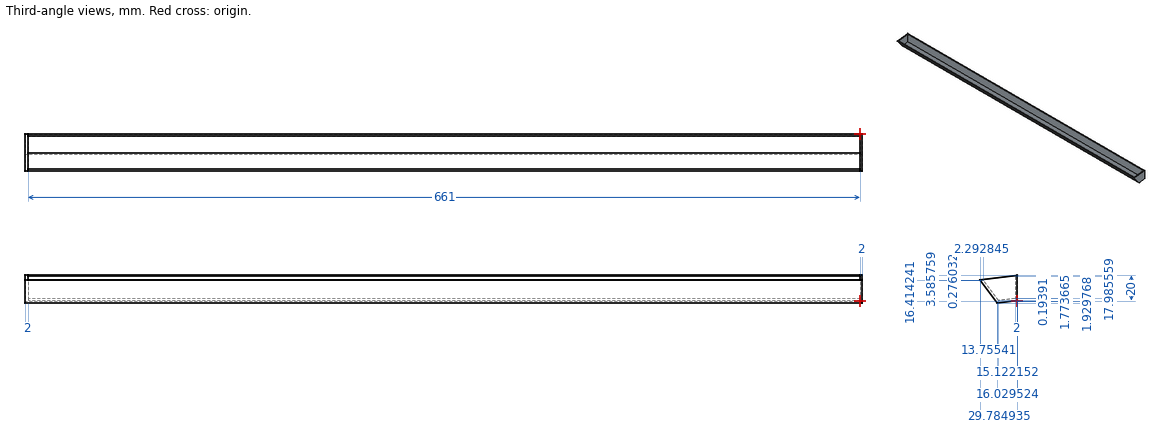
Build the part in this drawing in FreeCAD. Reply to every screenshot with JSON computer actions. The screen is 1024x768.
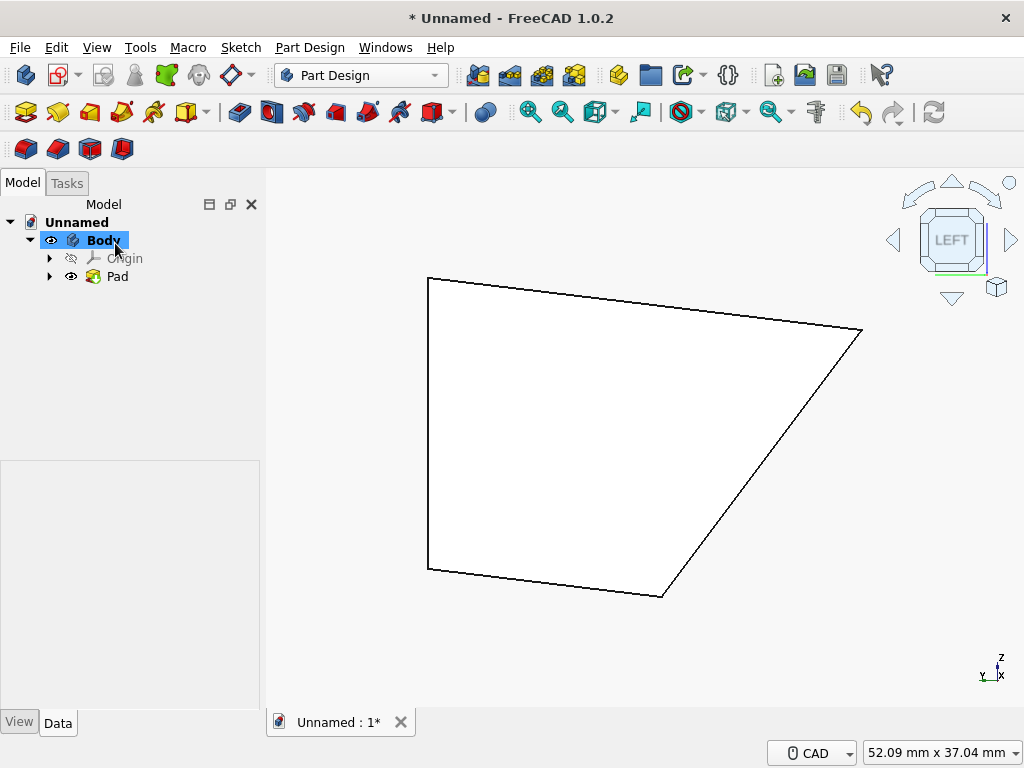
{"action": "left_click", "coordinate": [583, 437]}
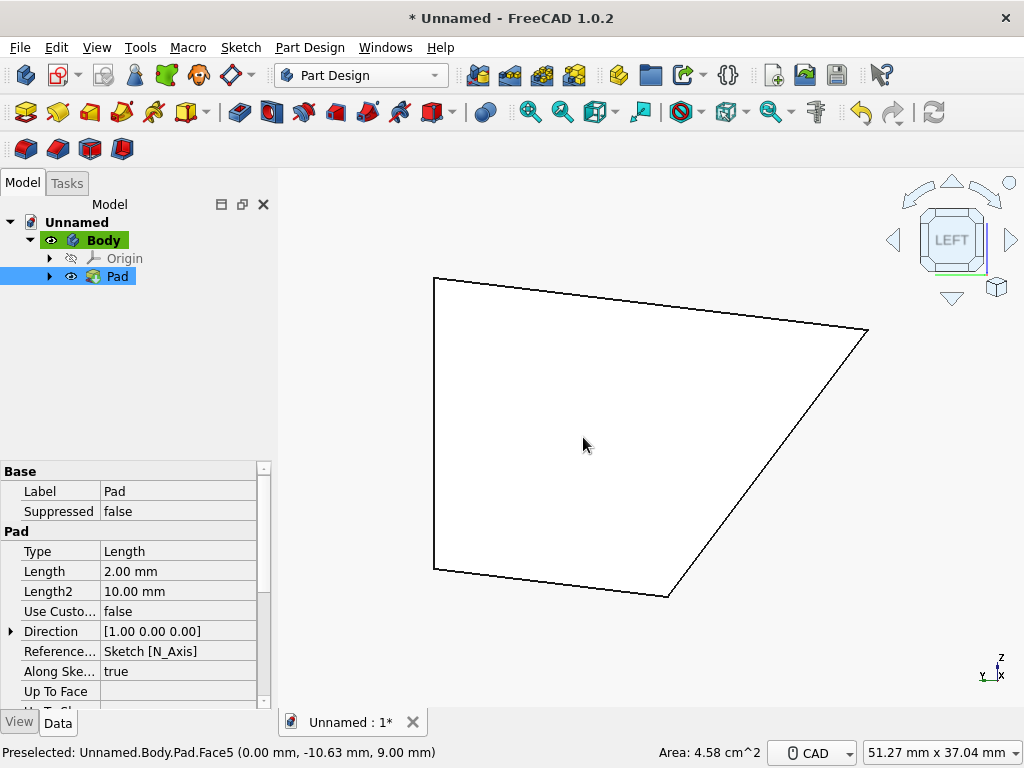
{"action": "left_click", "coordinate": [58, 76]}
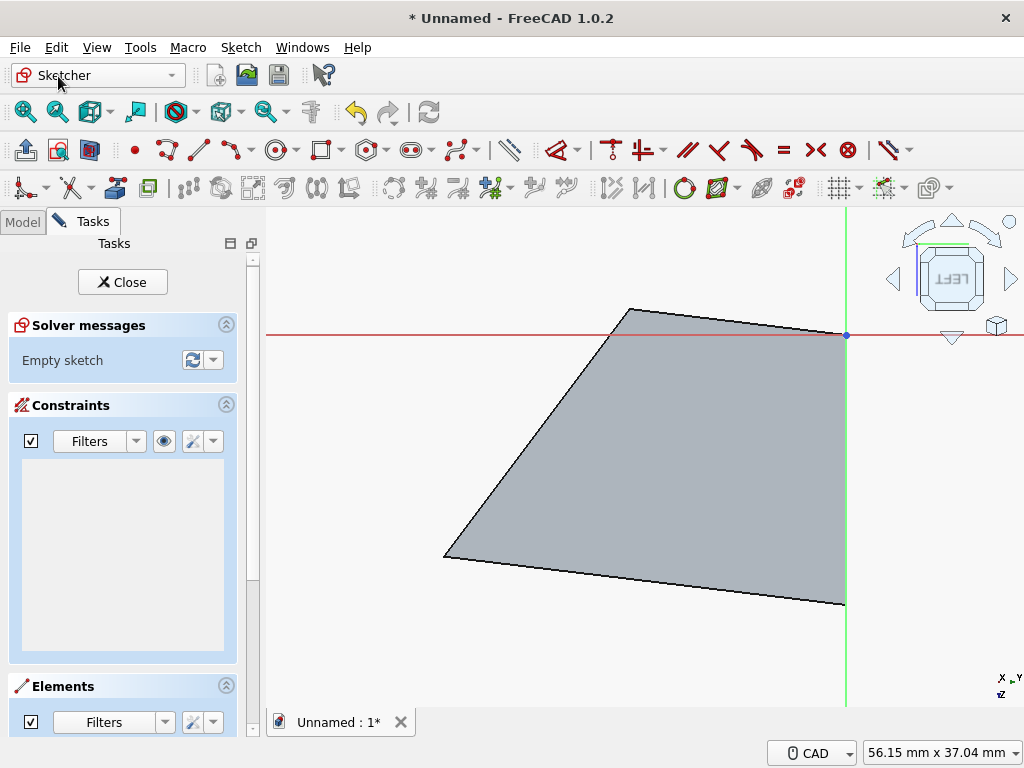
{"action": "scroll", "coordinate": [294, 457], "scroll_direction": "down", "scroll_amount": 1}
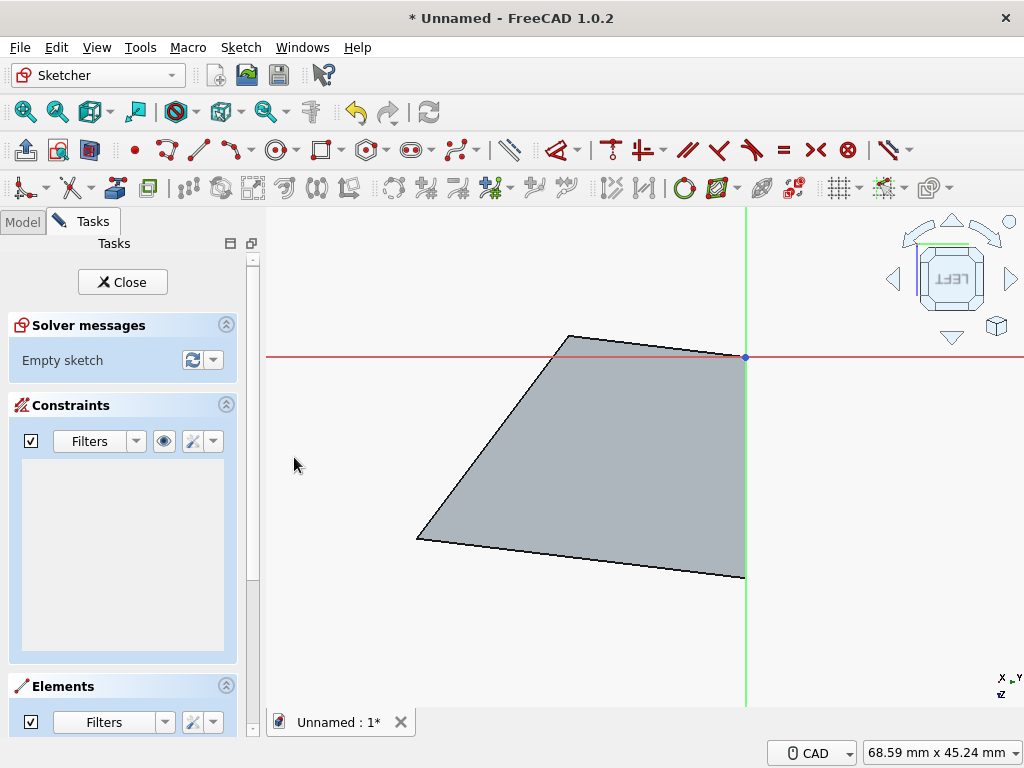
{"action": "left_click", "coordinate": [168, 150]}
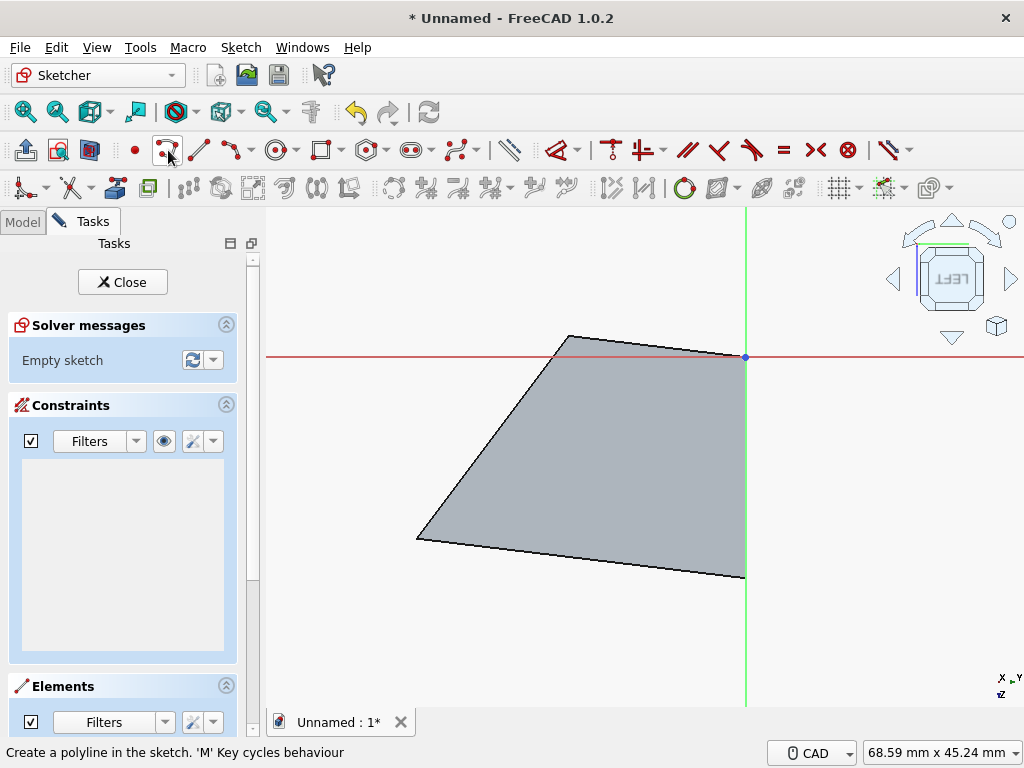
{"action": "left_click", "coordinate": [746, 357]}
{"action": "left_click", "coordinate": [569, 336]}
{"action": "left_click", "coordinate": [417, 539]}
{"action": "left_click", "coordinate": [442, 542]}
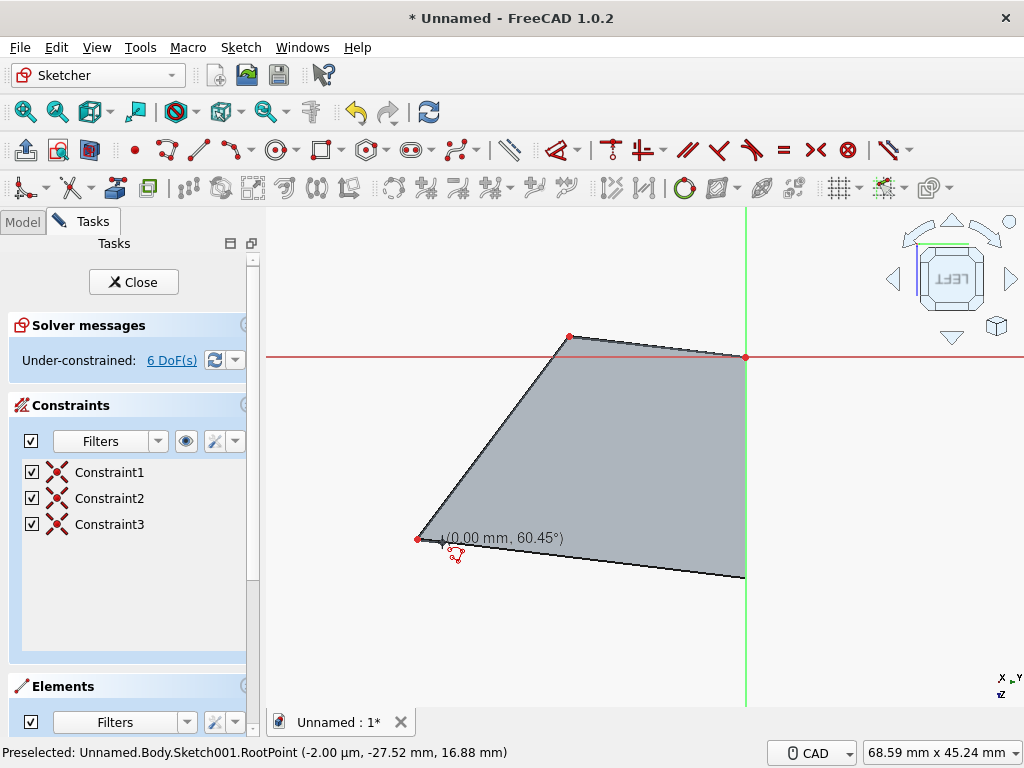
{"action": "scroll", "coordinate": [579, 359], "scroll_direction": "up", "scroll_amount": 11}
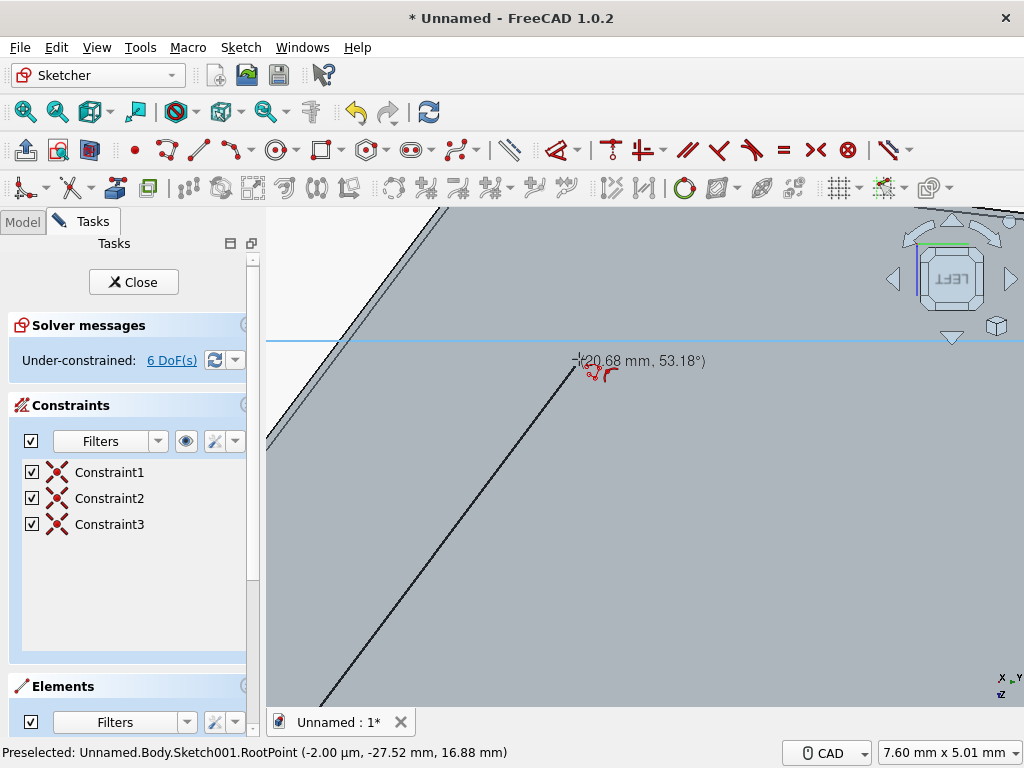
{"action": "left_click", "coordinate": [574, 360]}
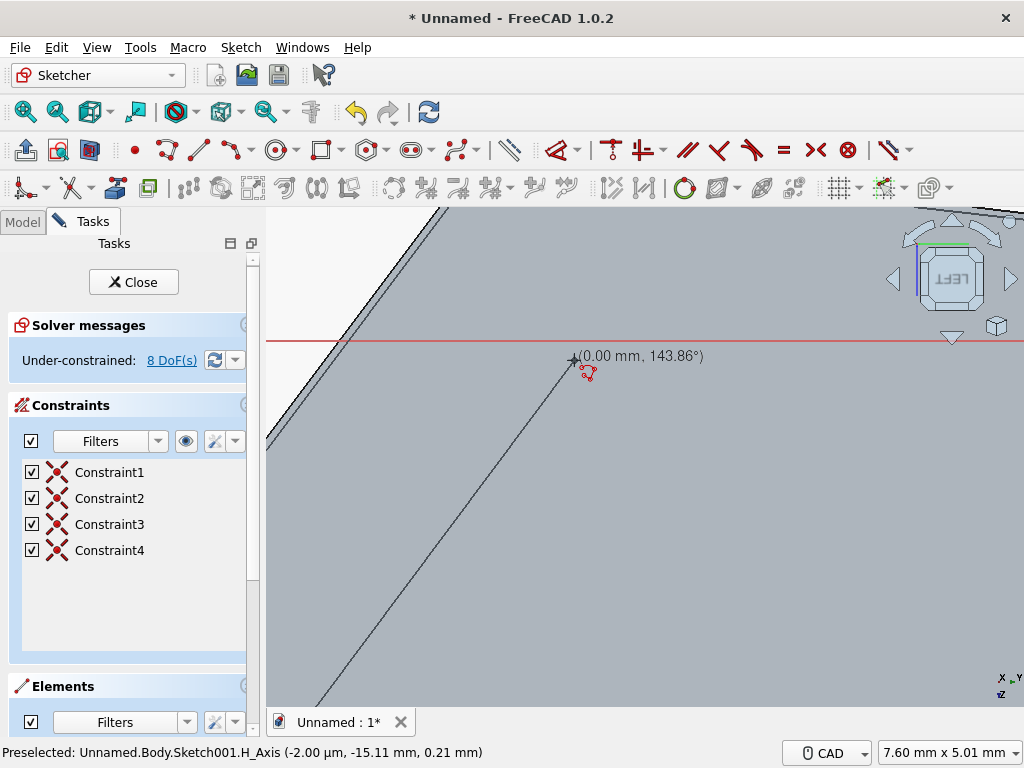
{"action": "scroll", "coordinate": [573, 334], "scroll_direction": "down", "scroll_amount": 10}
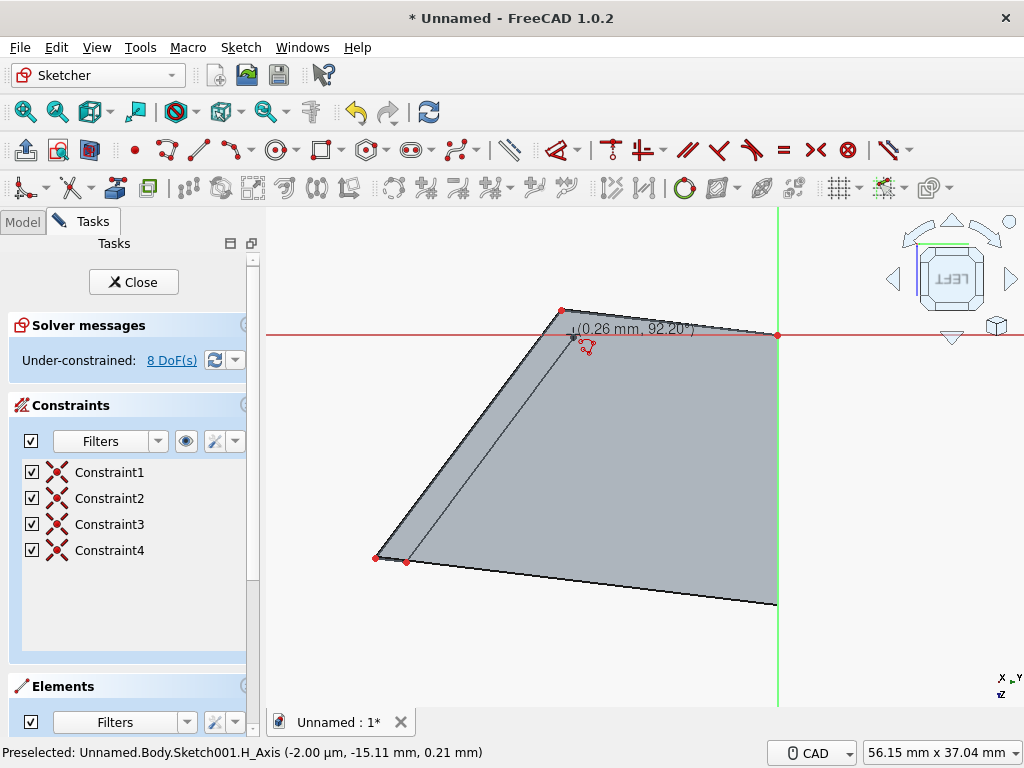
{"action": "left_click", "coordinate": [751, 359]}
{"action": "left_click", "coordinate": [751, 602]}
{"action": "left_click", "coordinate": [769, 605]}
{"action": "left_click", "coordinate": [778, 335]}
{"action": "key", "text": "Escape"}
{"action": "key", "text": "Escape"}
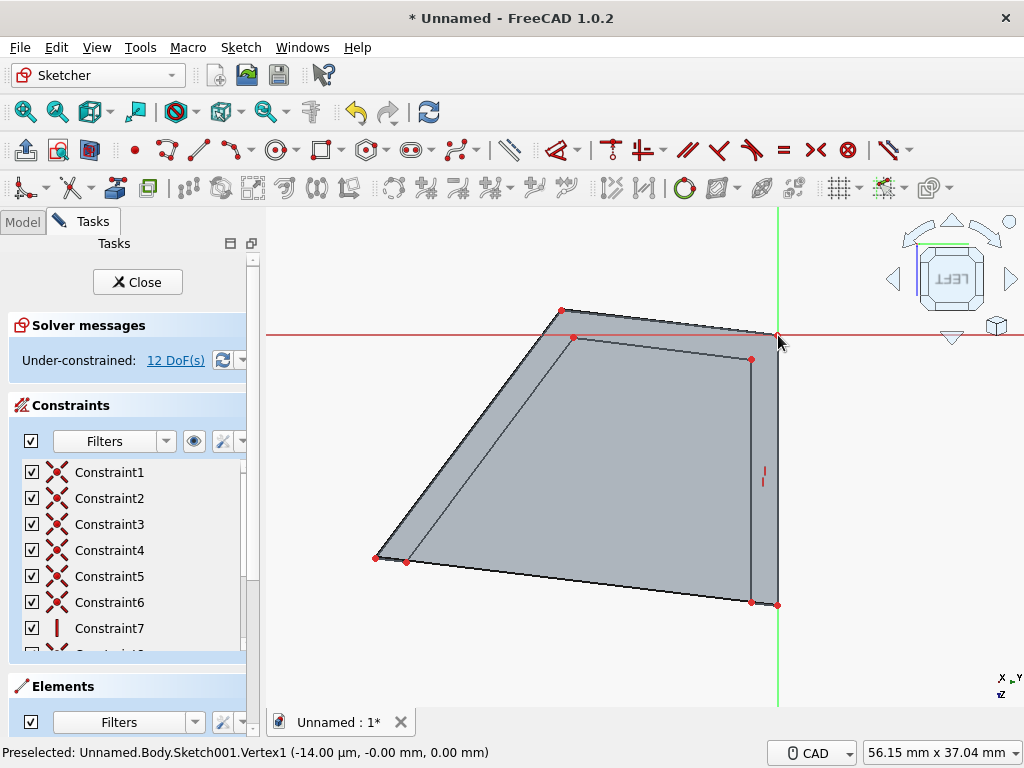
{"action": "left_click", "coordinate": [556, 150]}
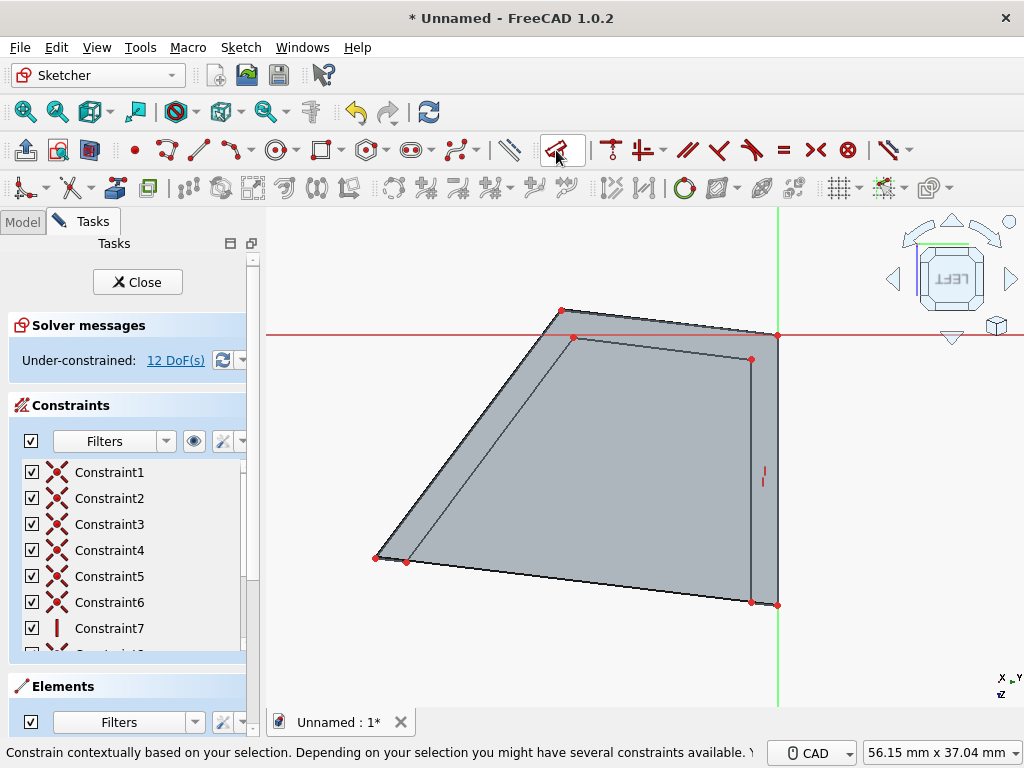
{"action": "left_click", "coordinate": [778, 525]}
{"action": "left_click", "coordinate": [812, 471]}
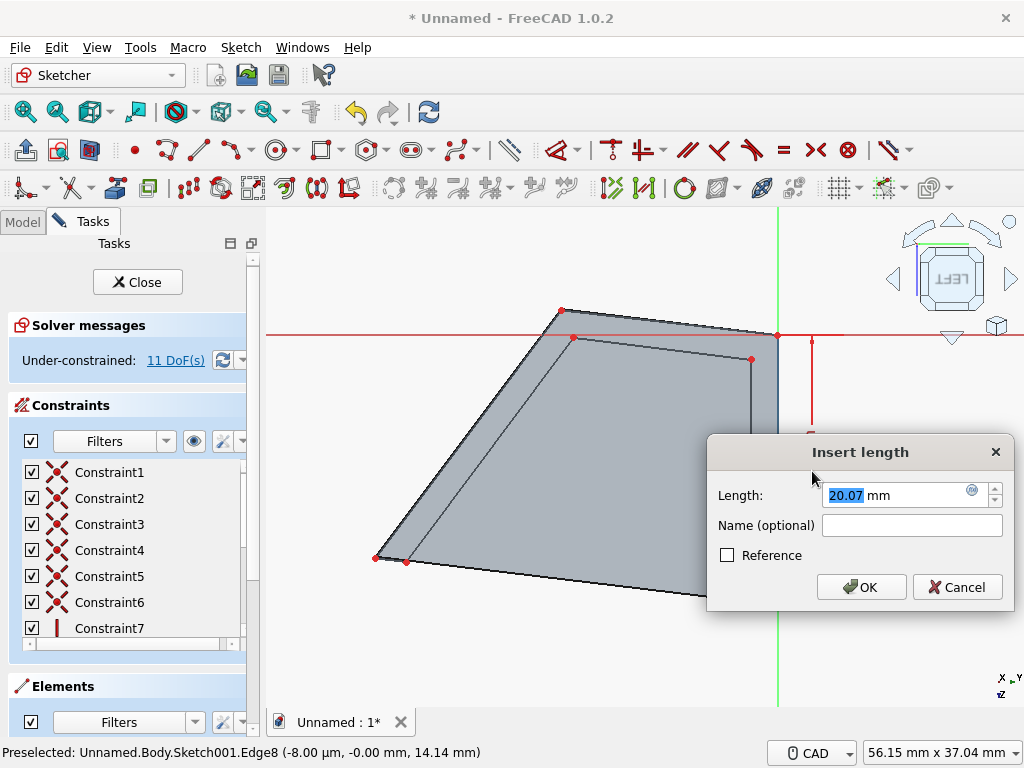
{"action": "type", "text": "20"}
{"action": "key", "text": "Return"}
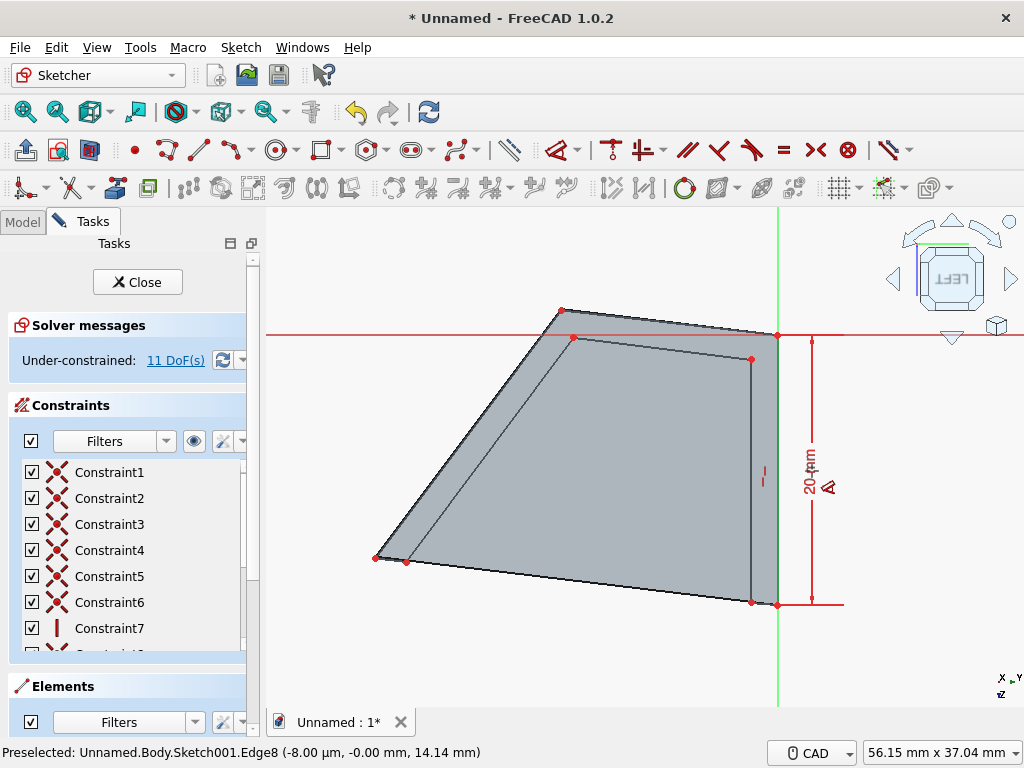
{"action": "scroll", "coordinate": [751, 360], "scroll_direction": "up", "scroll_amount": 2}